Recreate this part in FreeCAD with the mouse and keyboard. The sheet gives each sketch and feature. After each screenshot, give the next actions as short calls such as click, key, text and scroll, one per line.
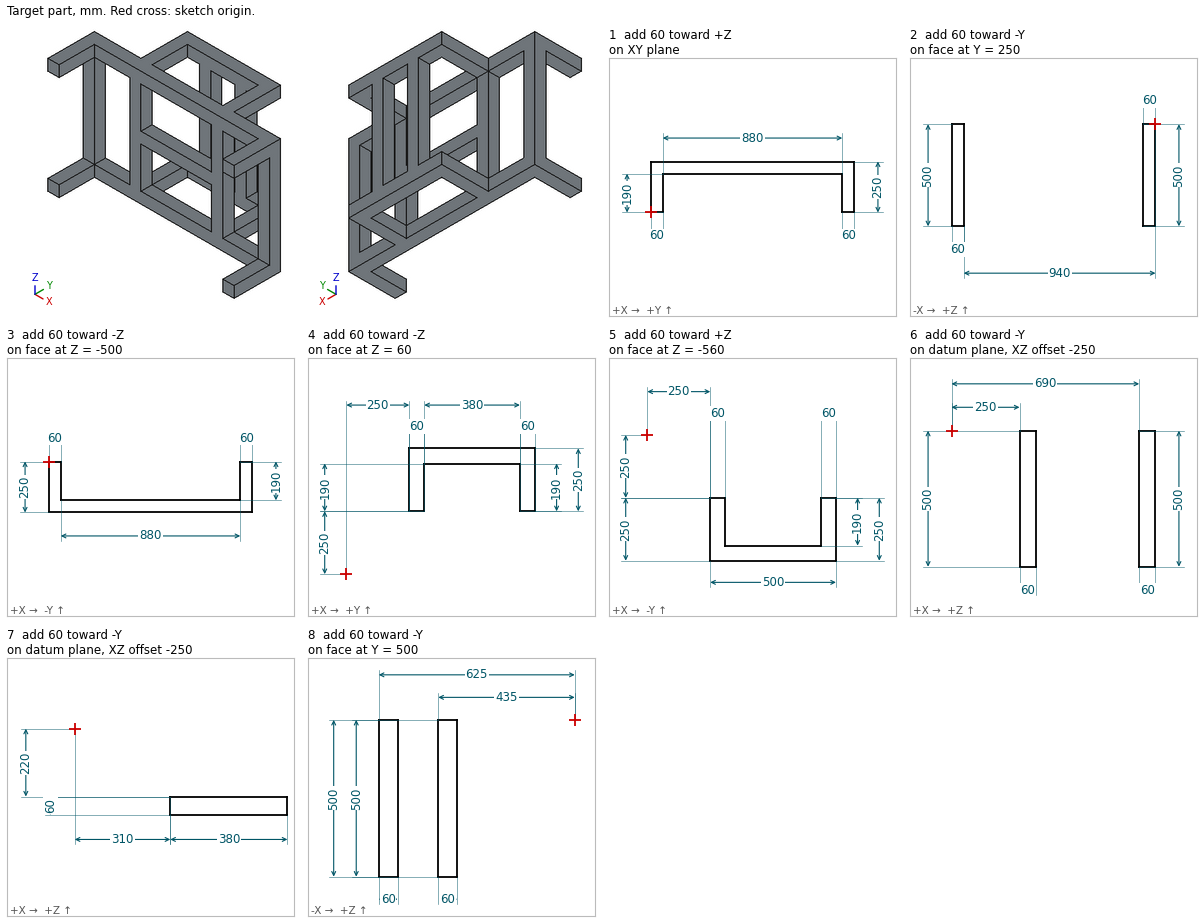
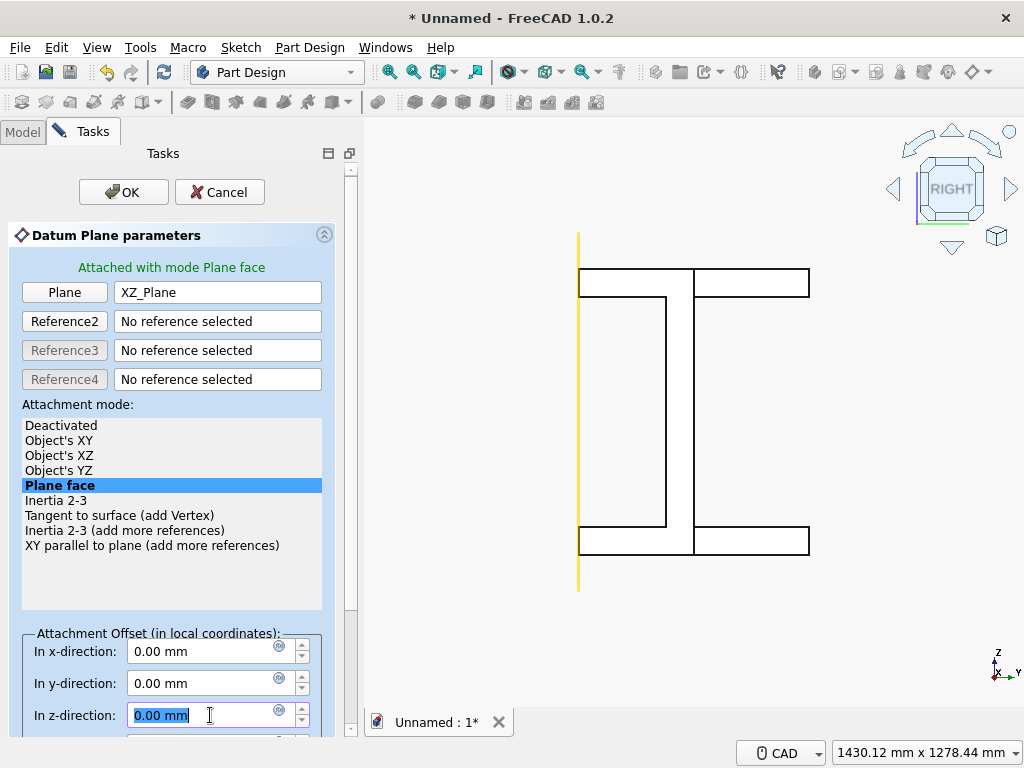
text(-250)
key(Tab)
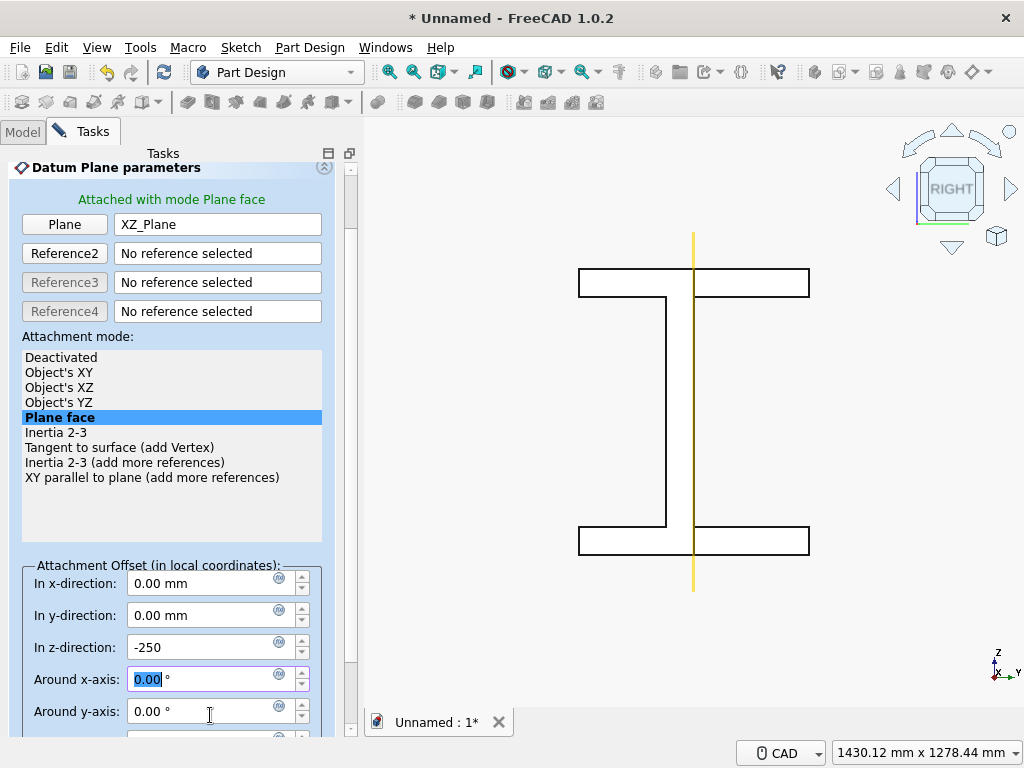
scroll(351, 450, up, 2)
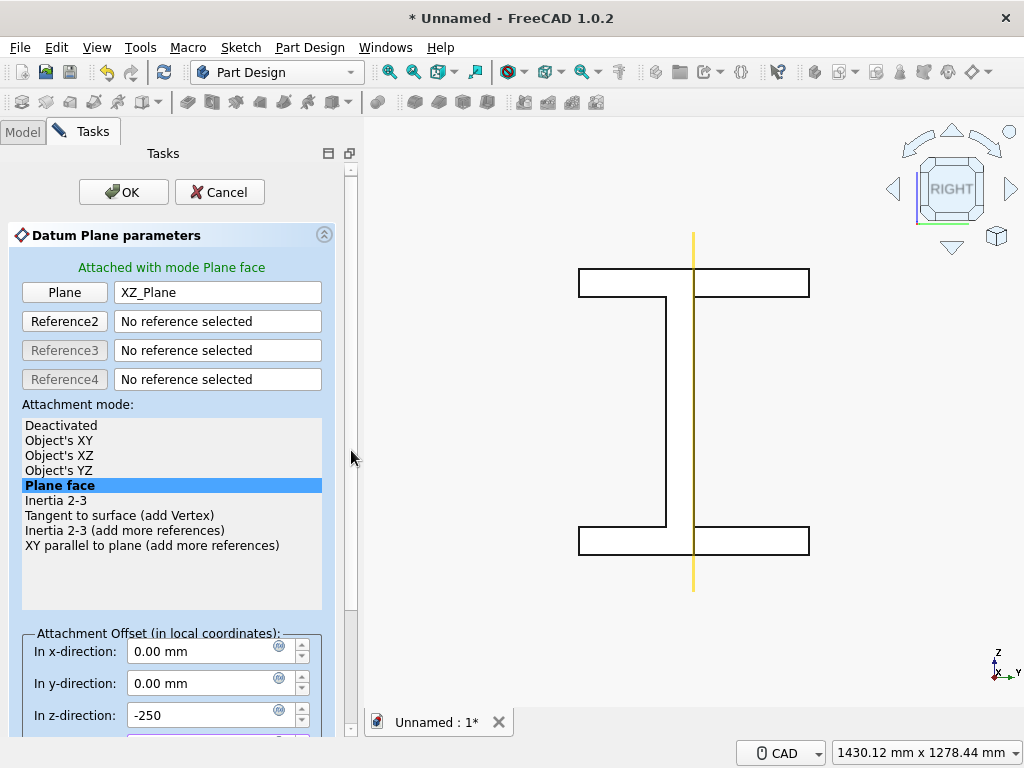
click(124, 192)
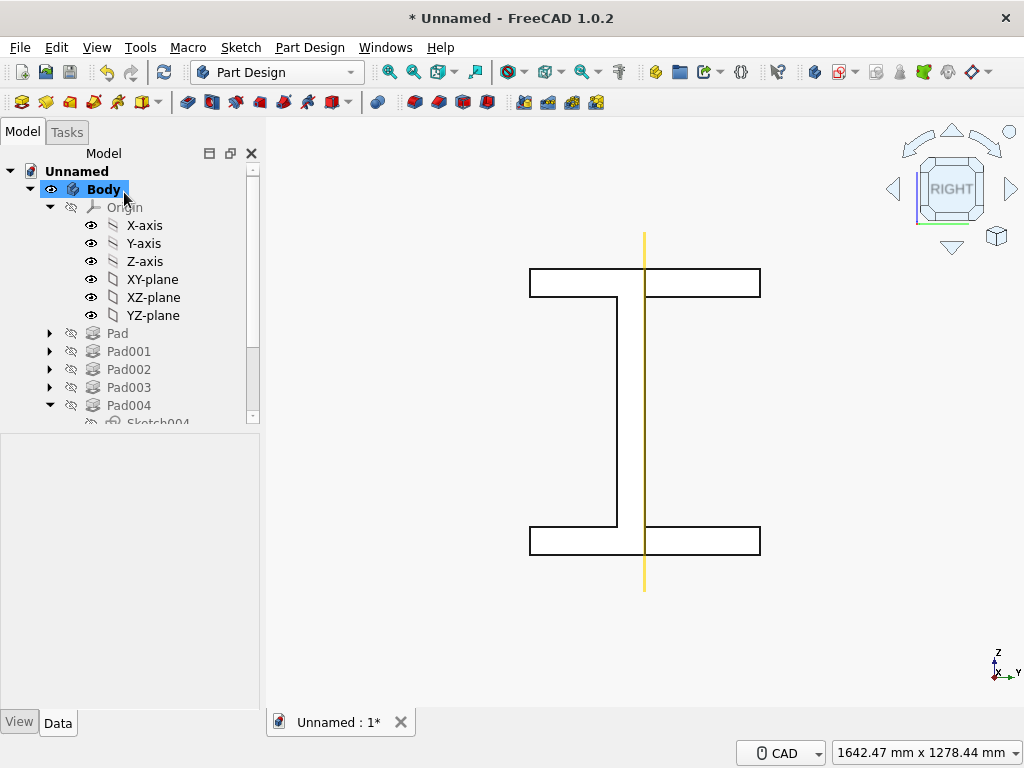
scroll(100, 293, down, 3)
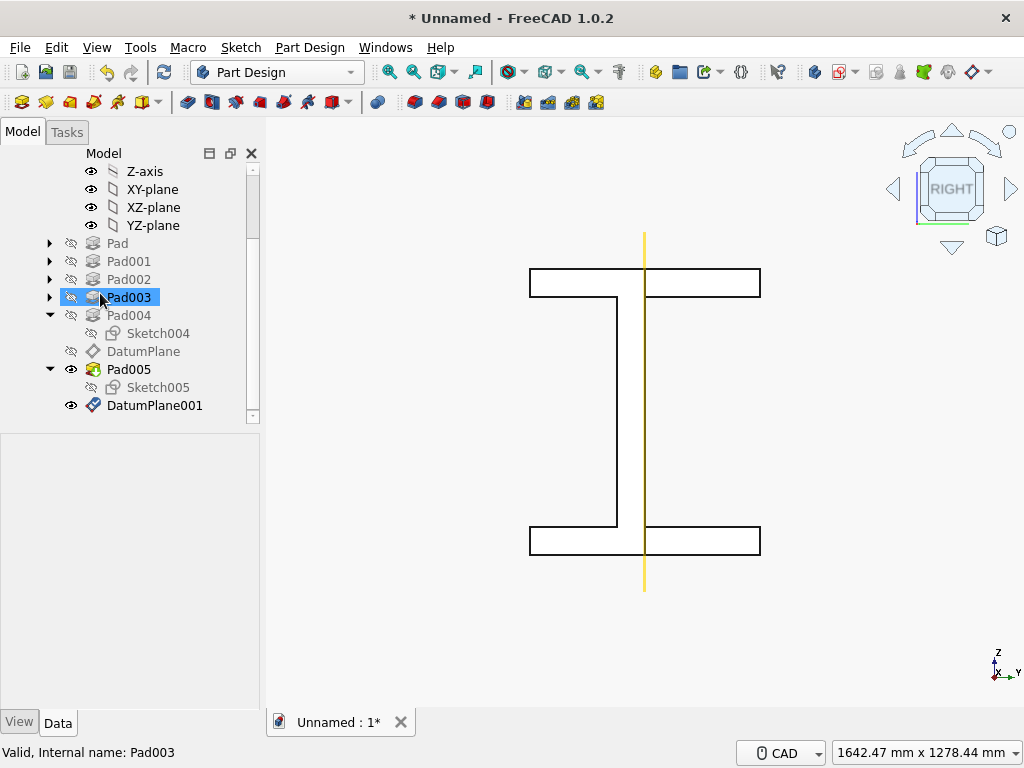
click(116, 405)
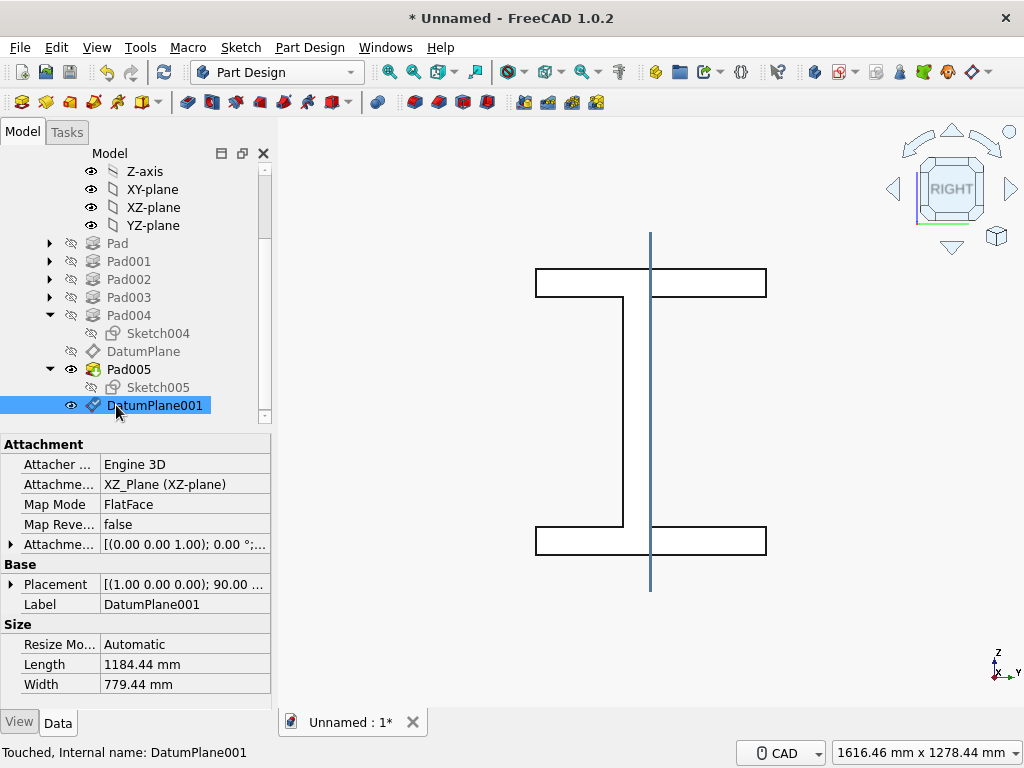
click(840, 72)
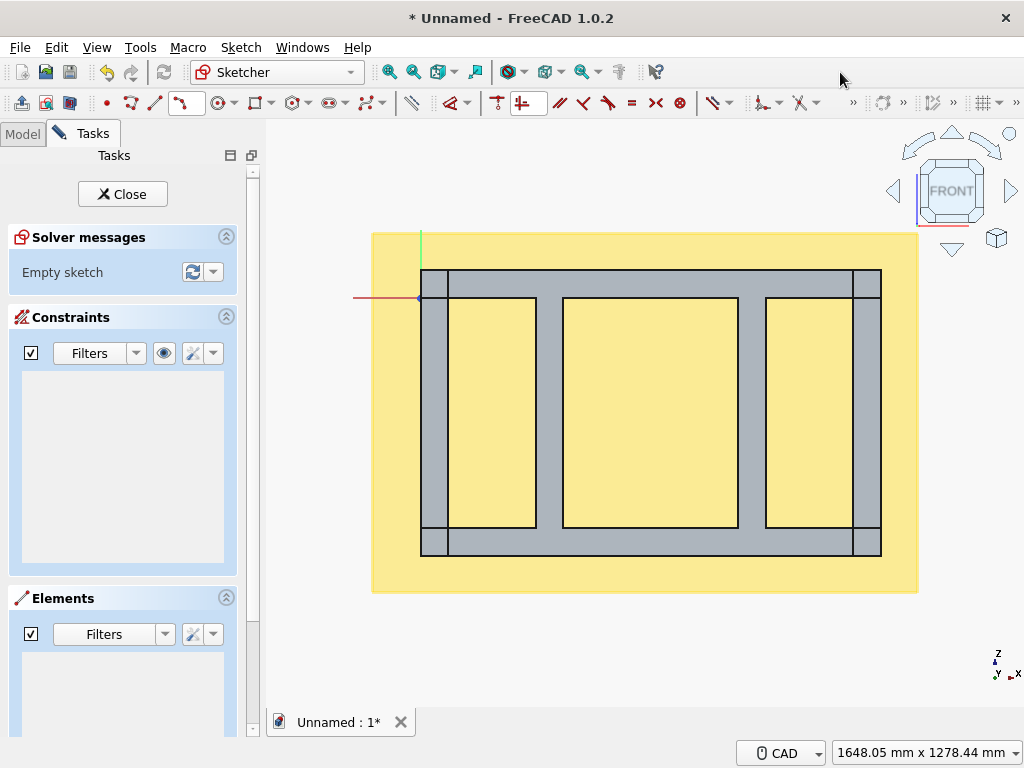
click(70, 104)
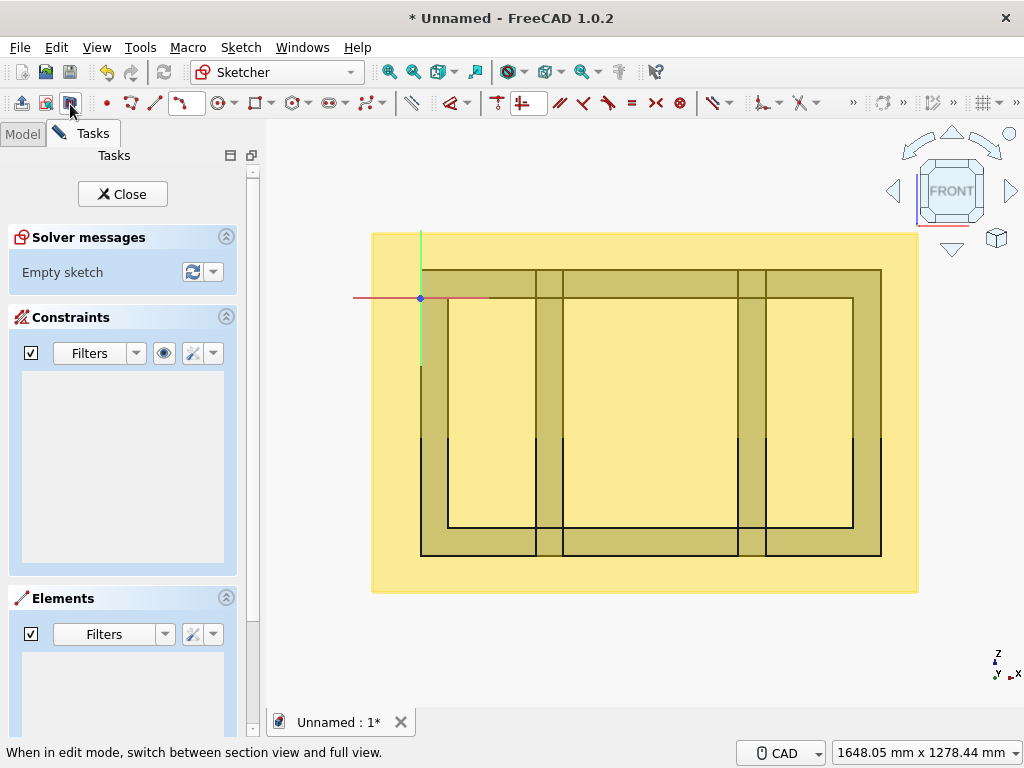
click(256, 104)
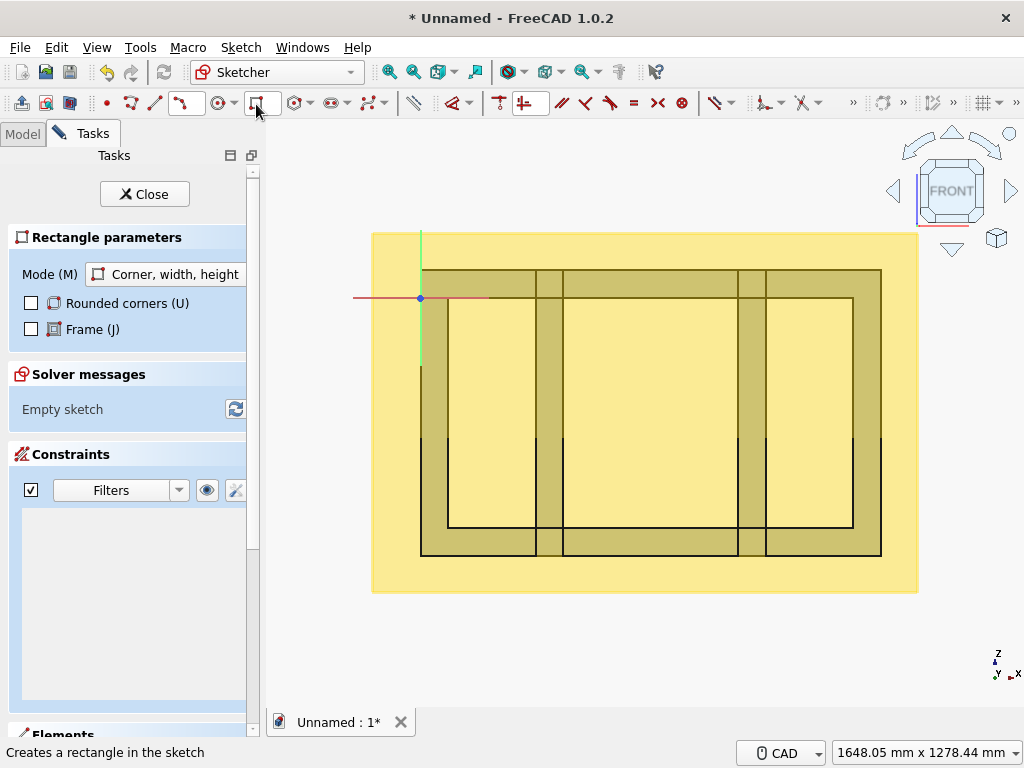
click(563, 399)
click(738, 427)
key(Escape)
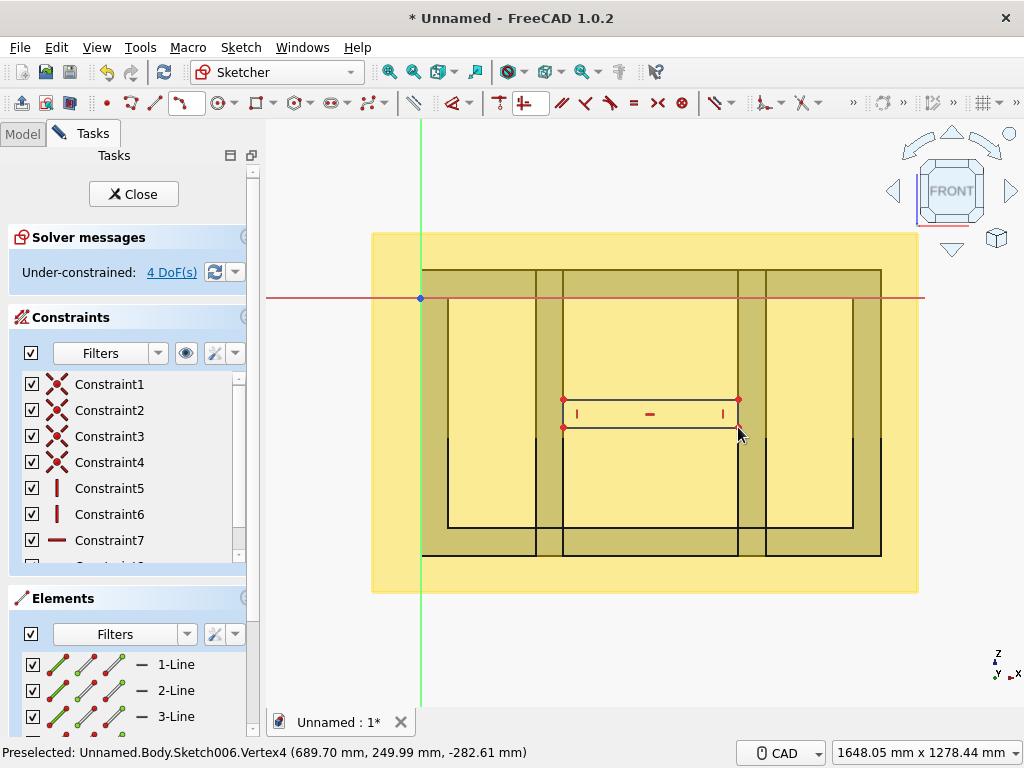
click(452, 104)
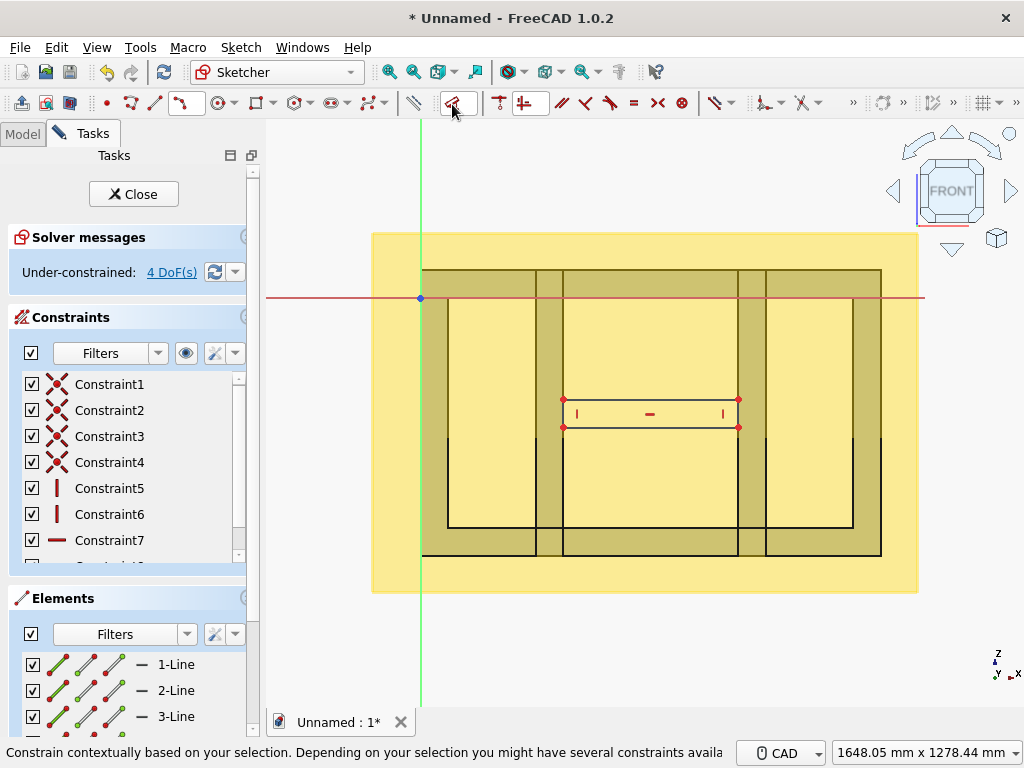
scroll(563, 411, up, 2)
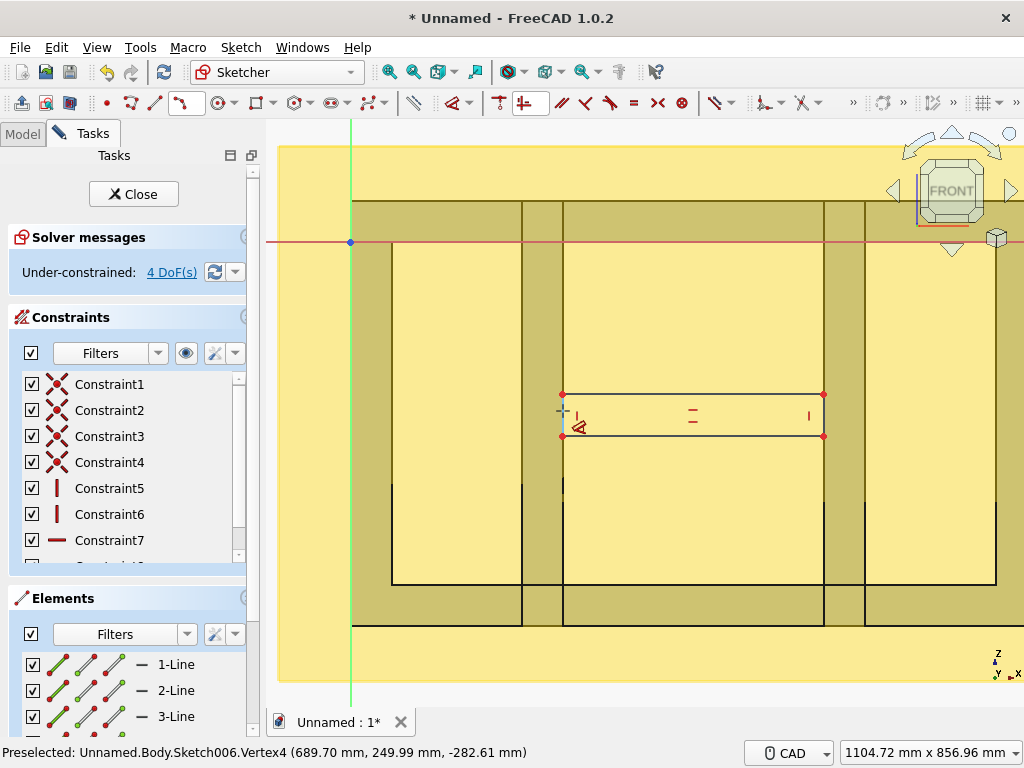
click(563, 411)
click(529, 415)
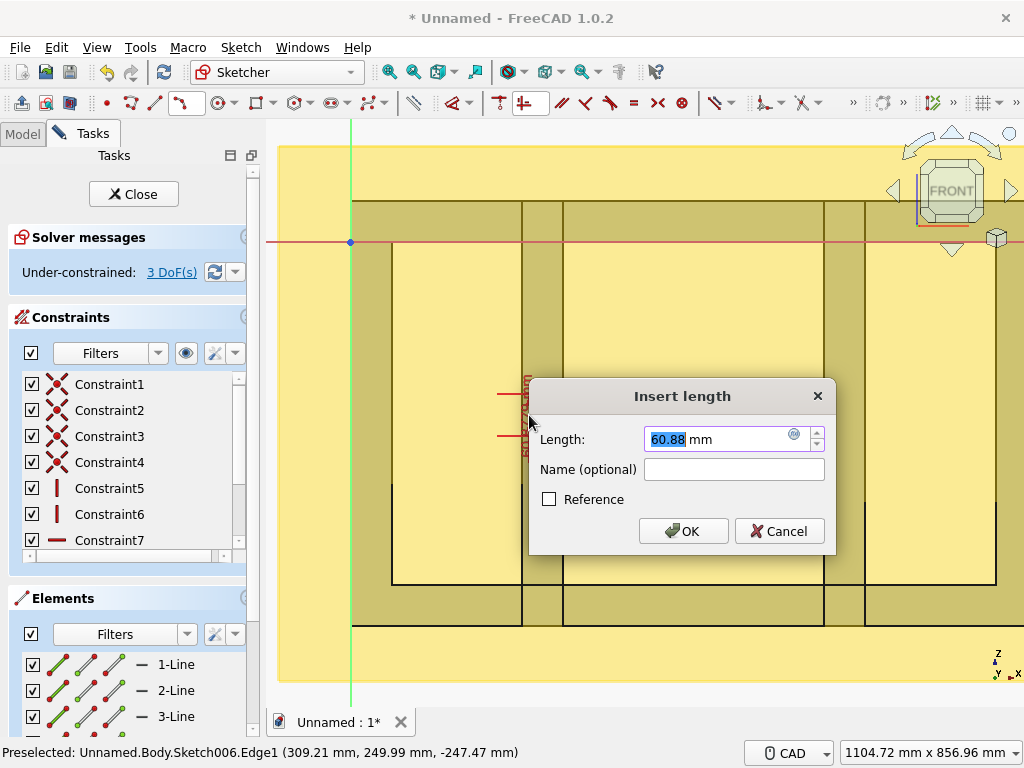
text(60)
key(Return)